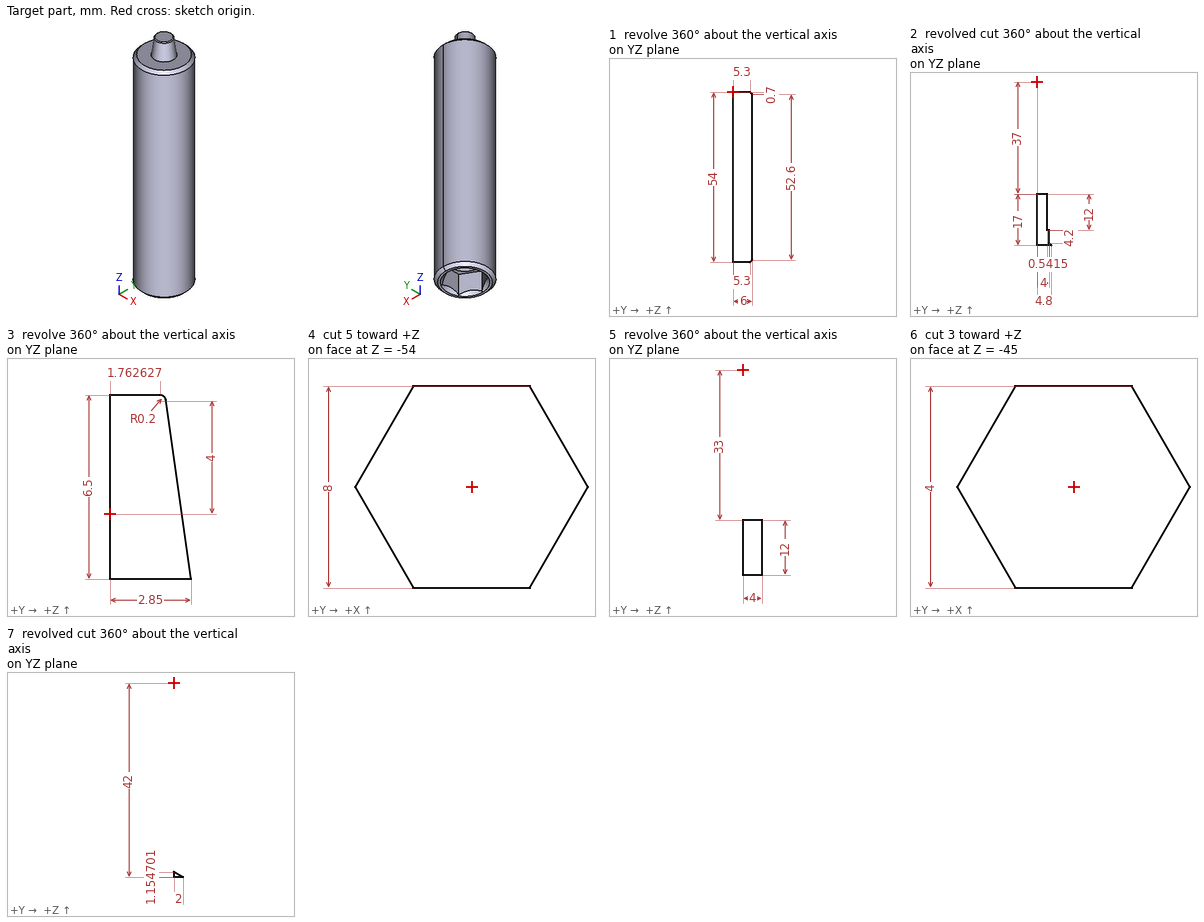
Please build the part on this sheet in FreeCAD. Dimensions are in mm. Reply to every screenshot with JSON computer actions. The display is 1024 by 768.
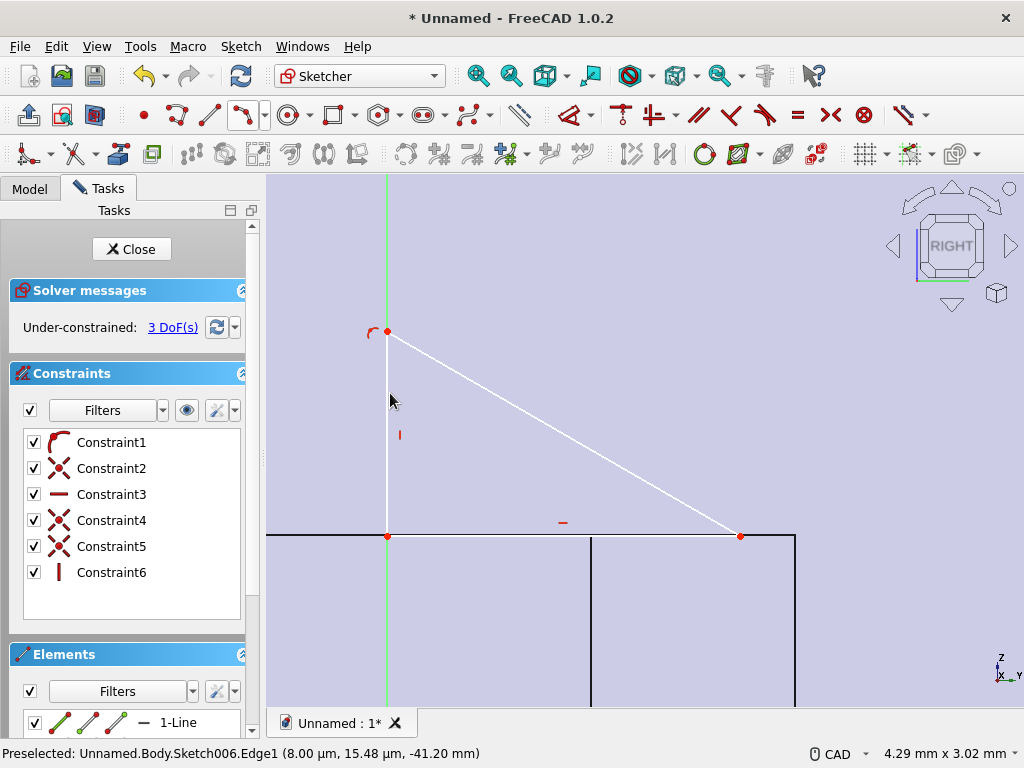
{"action": "left_click", "coordinate": [568, 116]}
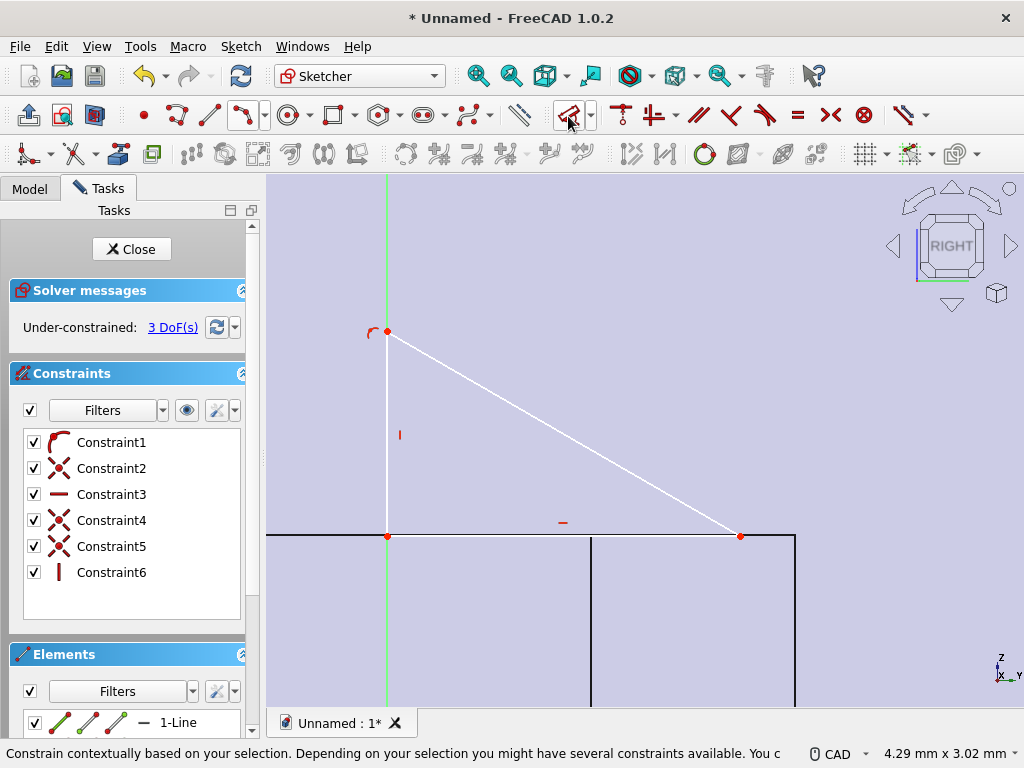
{"action": "left_click", "coordinate": [493, 536]}
{"action": "left_click", "coordinate": [564, 570]}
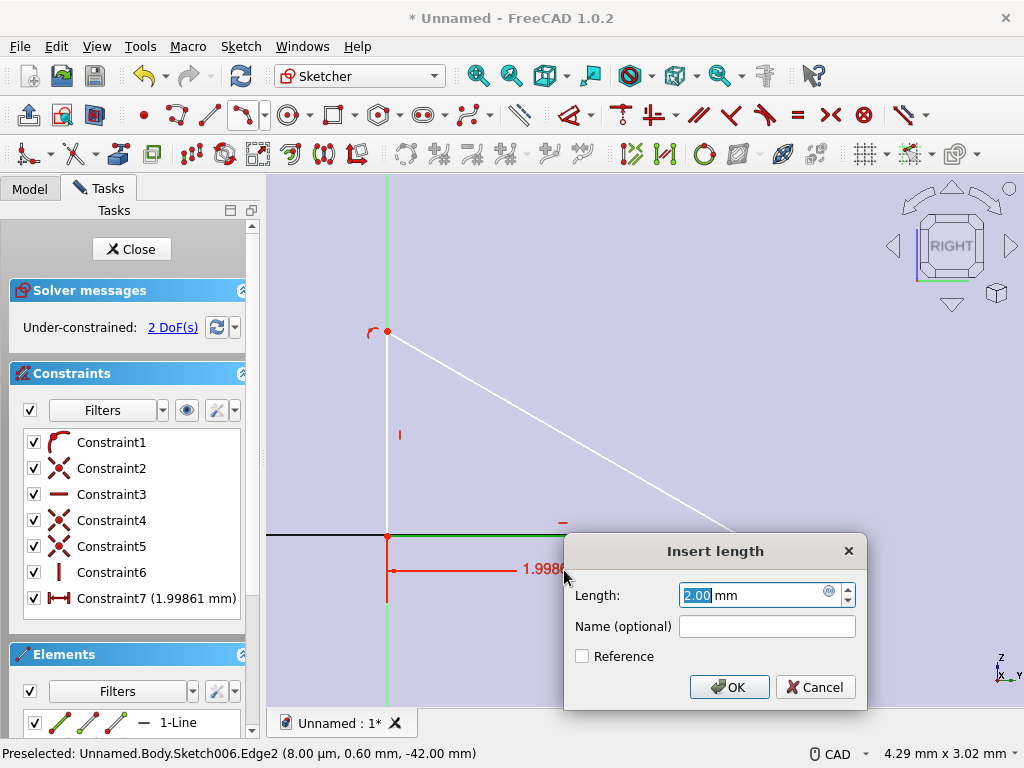
{"action": "type", "text": "2"}
{"action": "key", "text": "Return"}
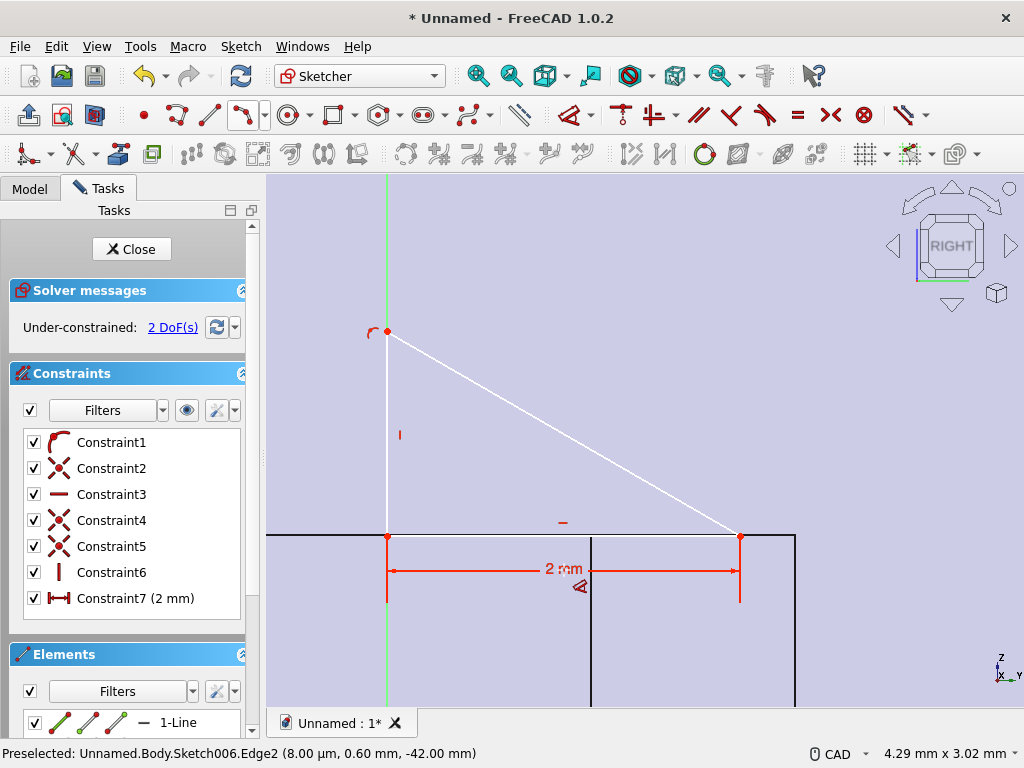
{"action": "left_click", "coordinate": [387, 536]}
{"action": "left_click", "coordinate": [353, 369]}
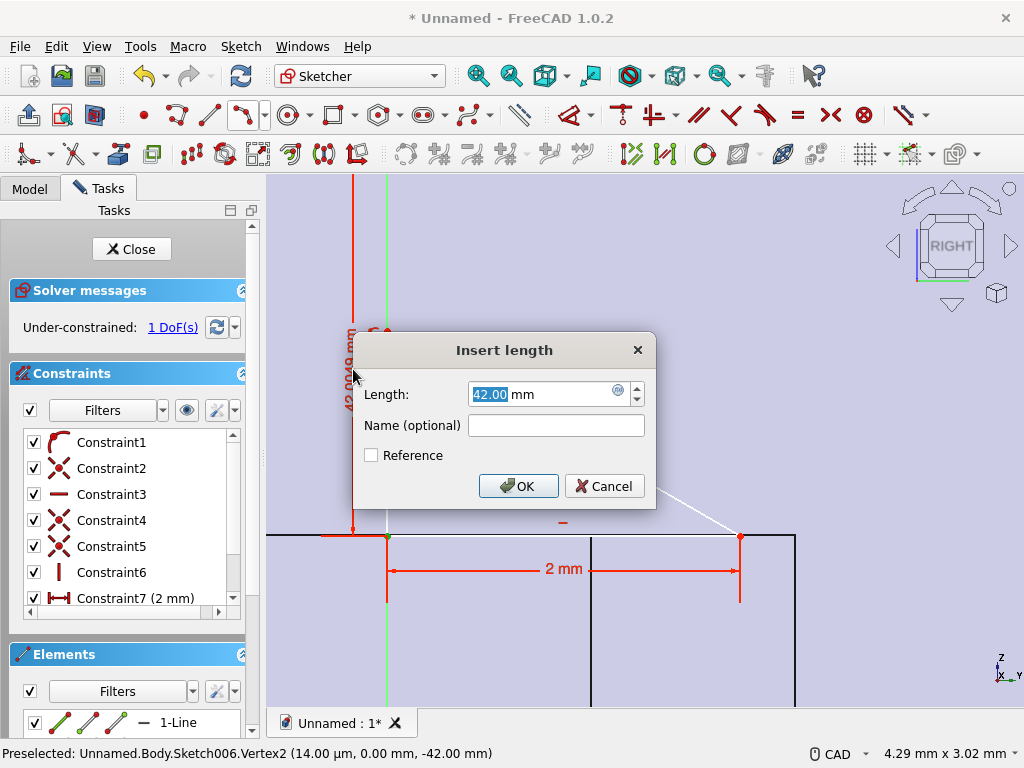
{"action": "type", "text": "42"}
{"action": "key", "text": "Return"}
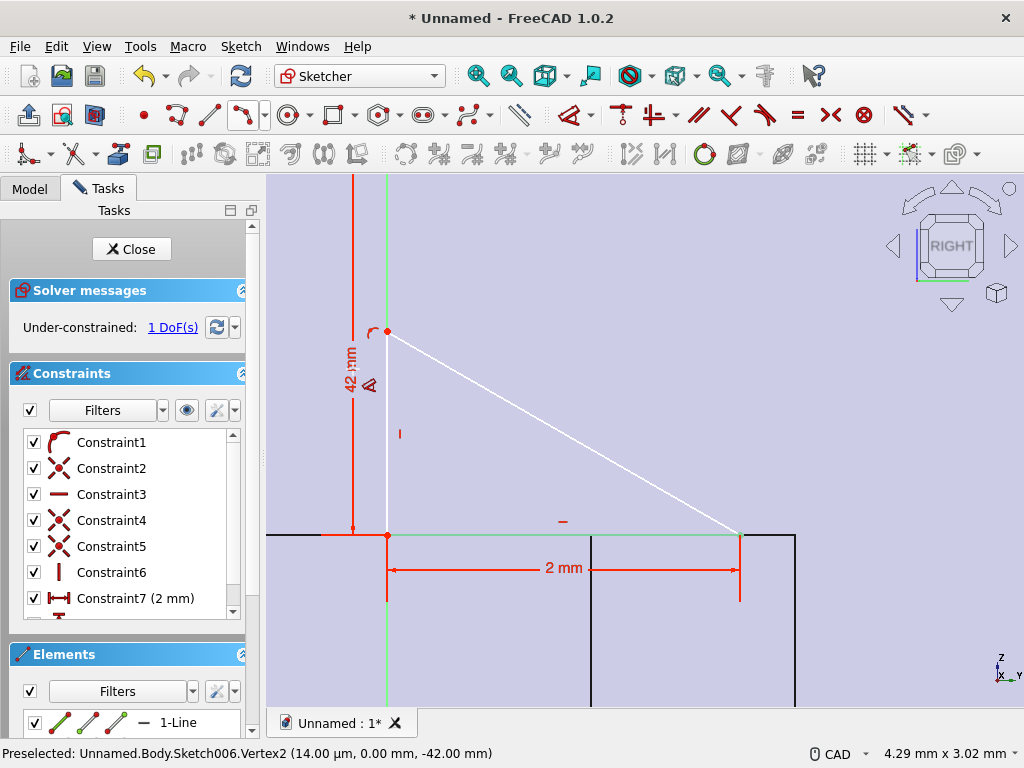
{"action": "left_click", "coordinate": [387, 393]}
{"action": "left_click", "coordinate": [353, 434]}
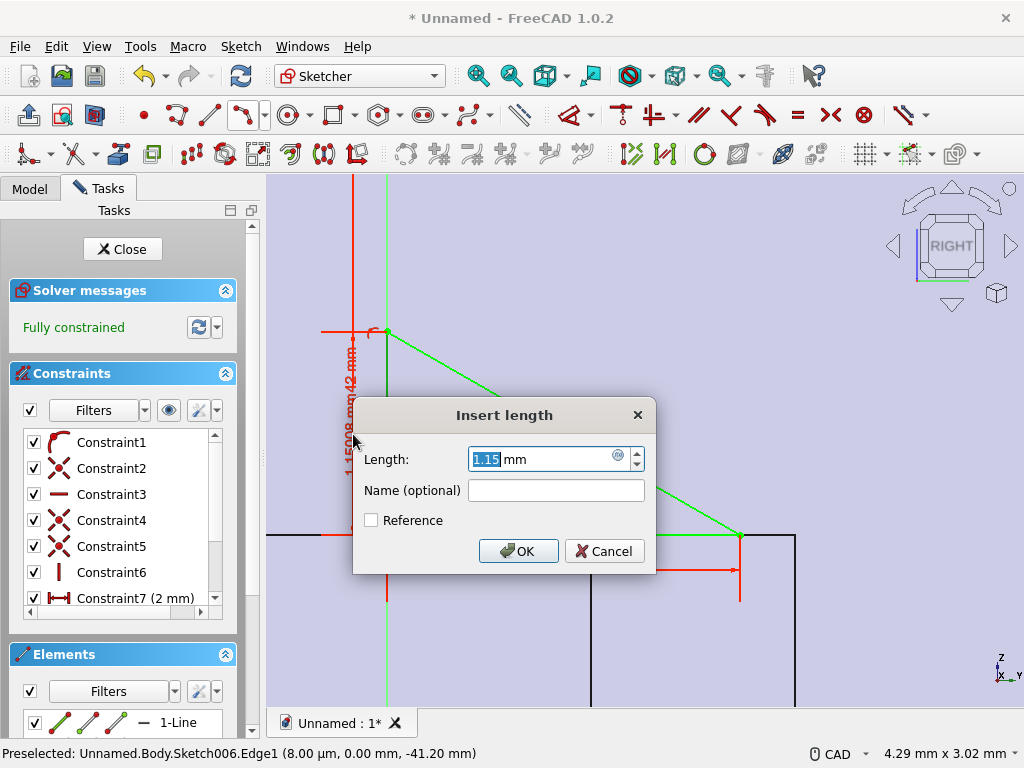
{"action": "type", "text": "1.154701"}
{"action": "key", "text": "Return"}
{"action": "key", "text": "Escape"}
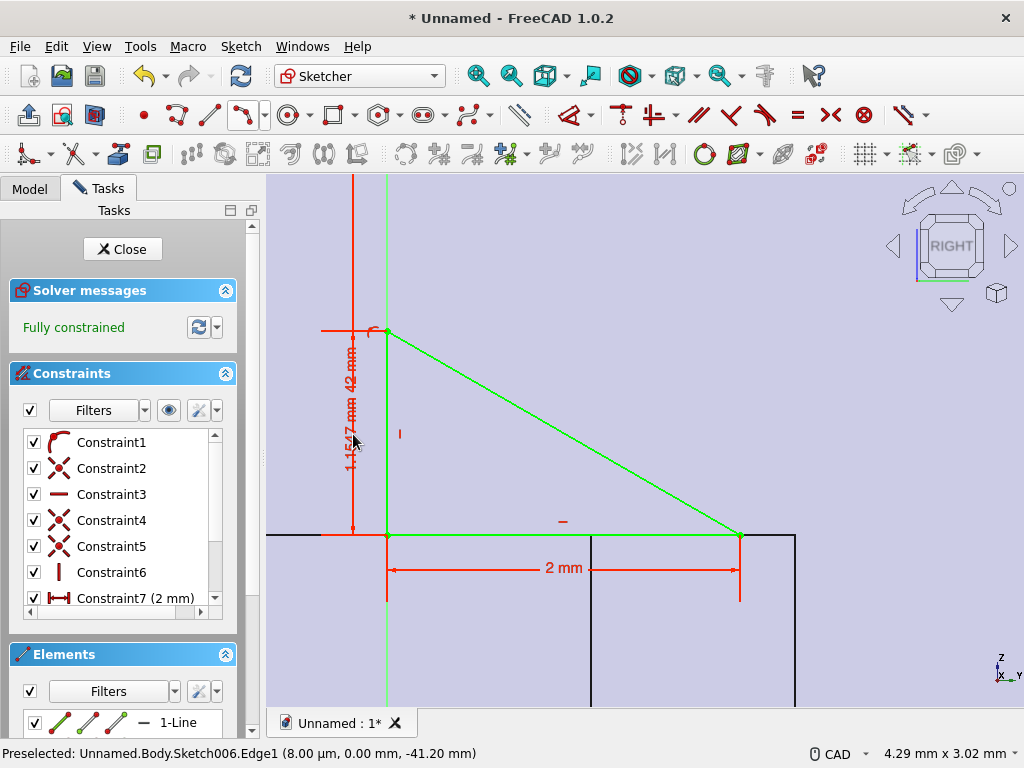
{"action": "left_click", "coordinate": [123, 249]}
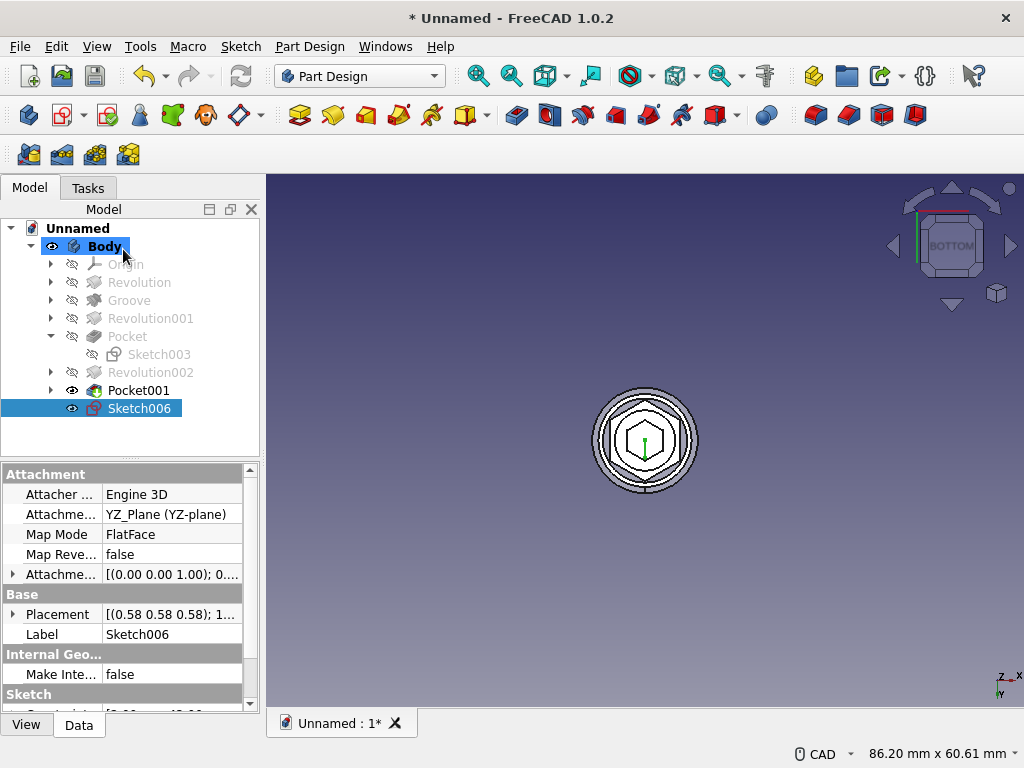
{"action": "left_click", "coordinate": [583, 116]}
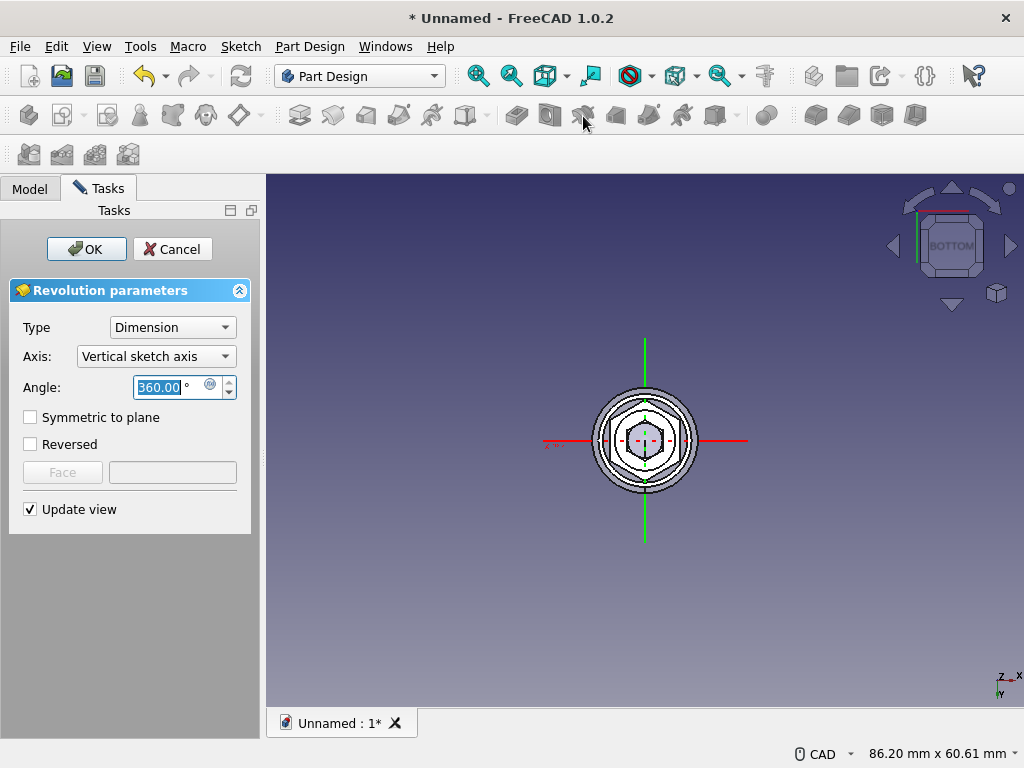
{"action": "left_click", "coordinate": [87, 249]}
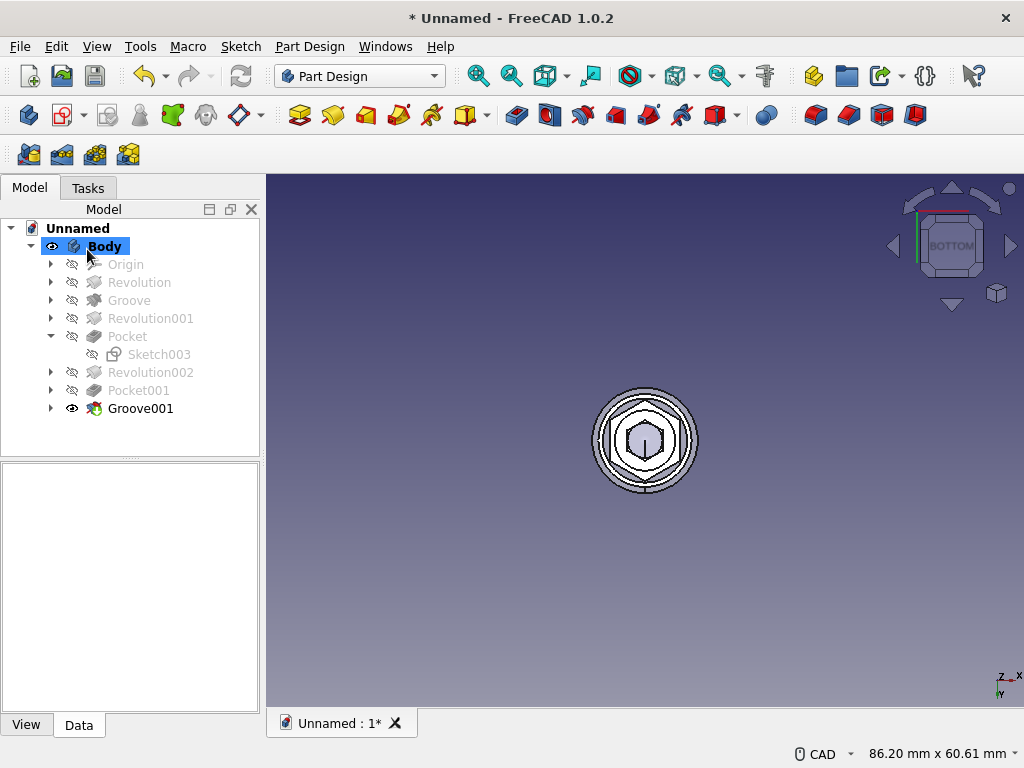
{"action": "key", "text": "0"}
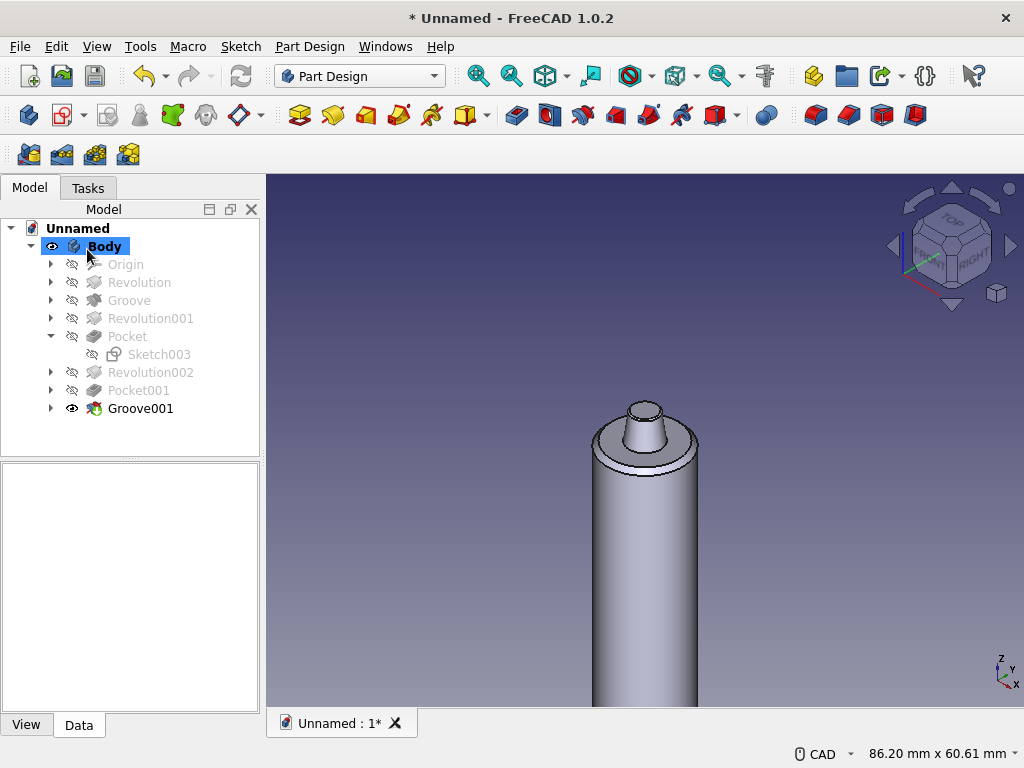
{"action": "left_click", "coordinate": [479, 76]}